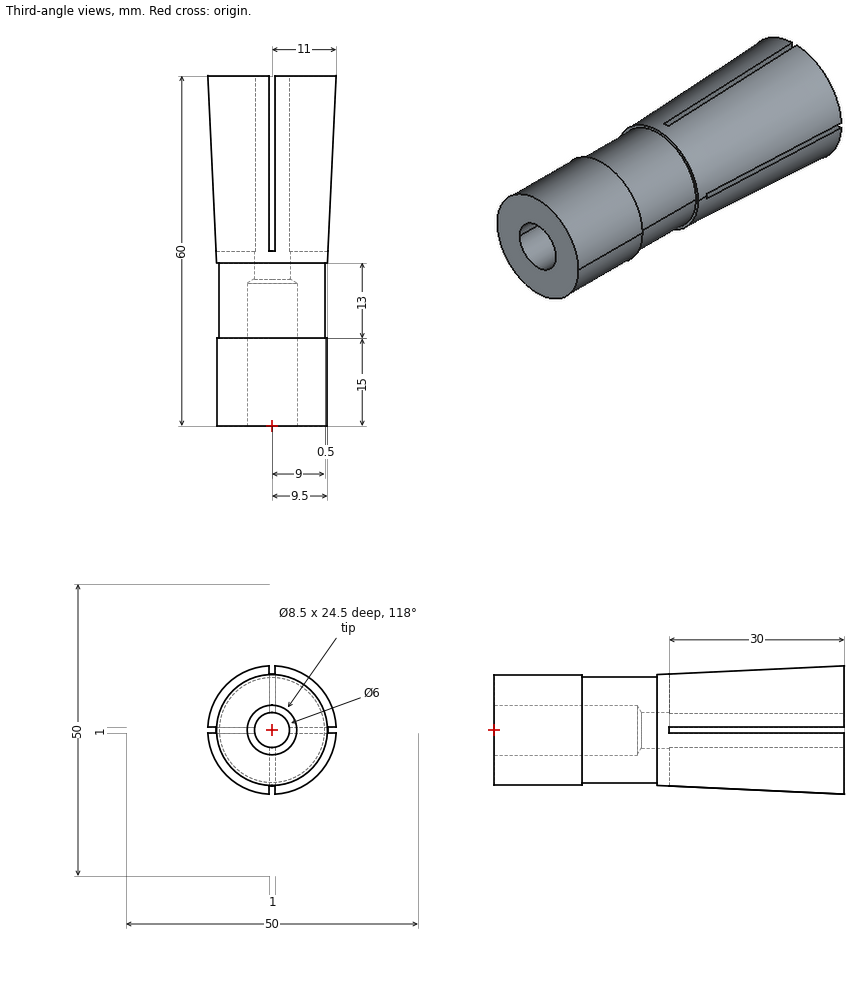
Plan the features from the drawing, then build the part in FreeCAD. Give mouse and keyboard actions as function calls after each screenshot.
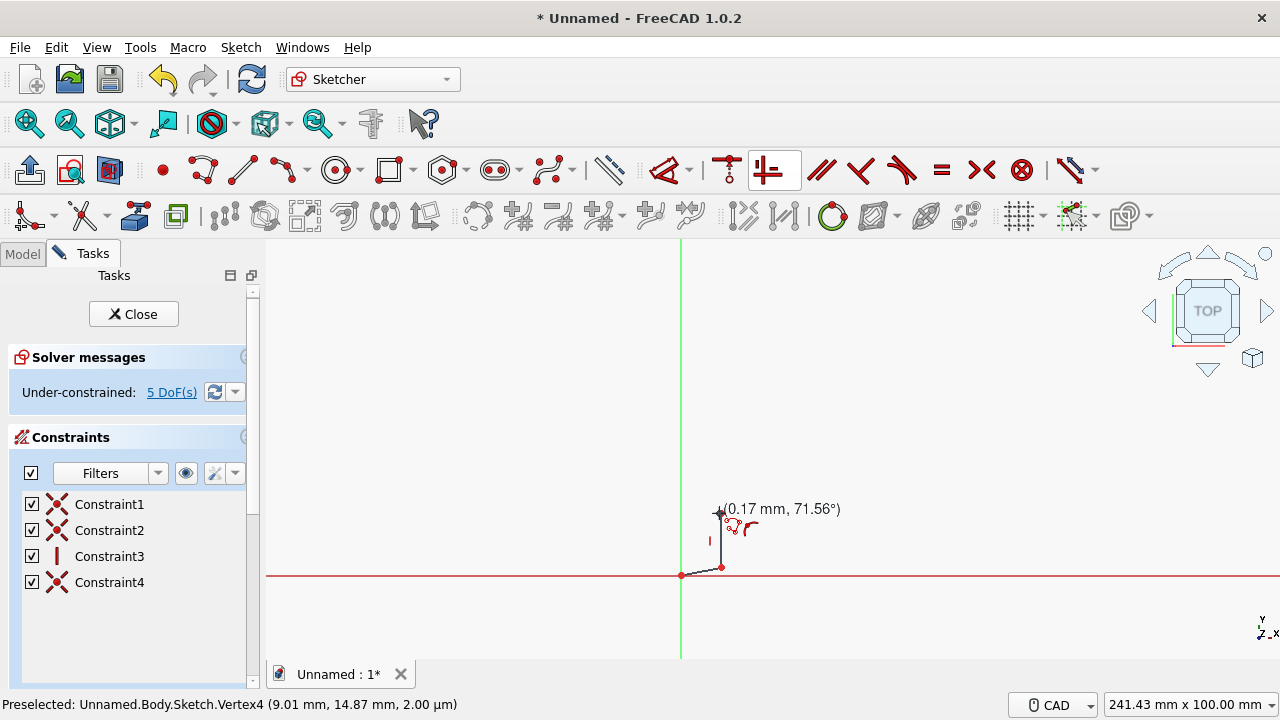
click(719, 458)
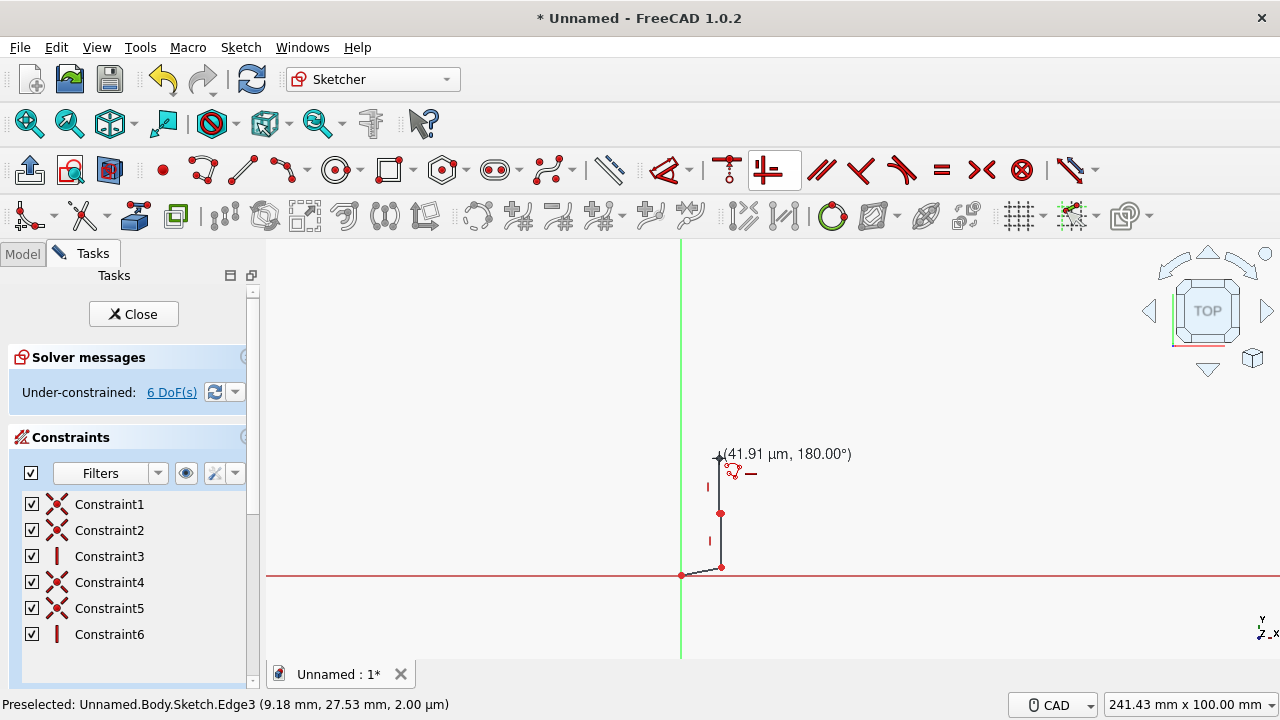
scroll(721, 458, up, 11)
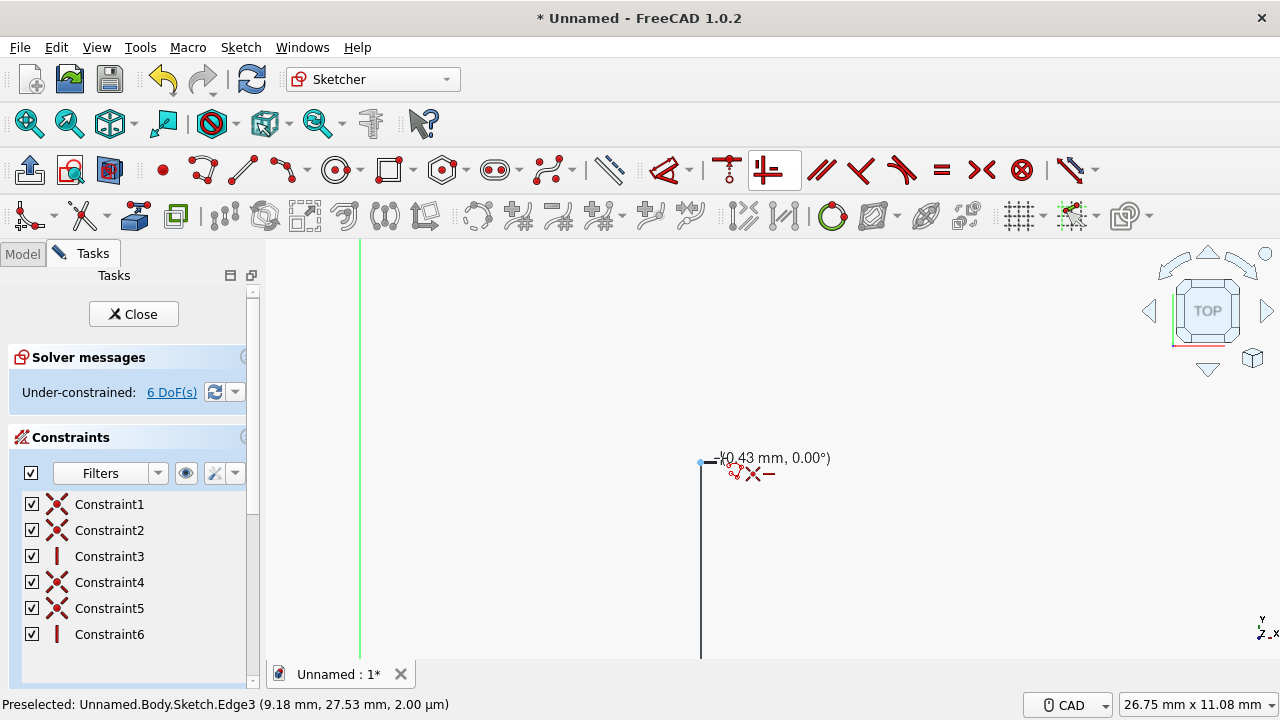
click(720, 454)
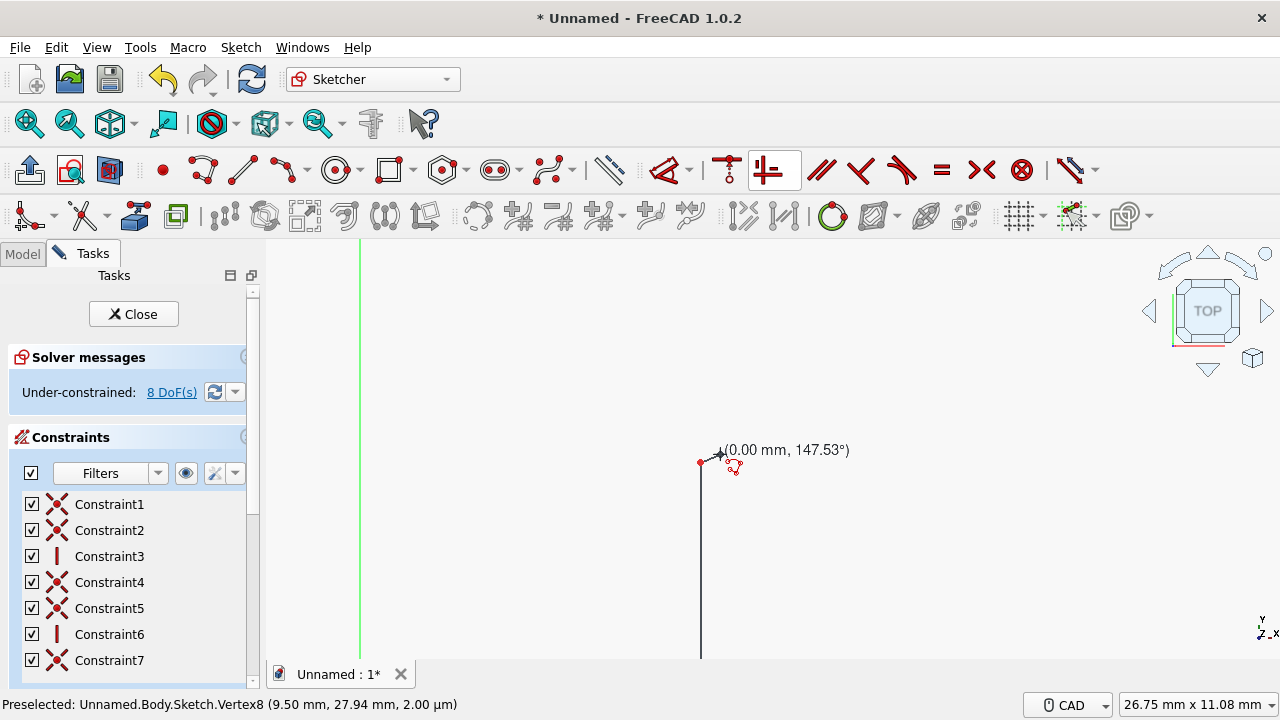
scroll(721, 458, down, 11)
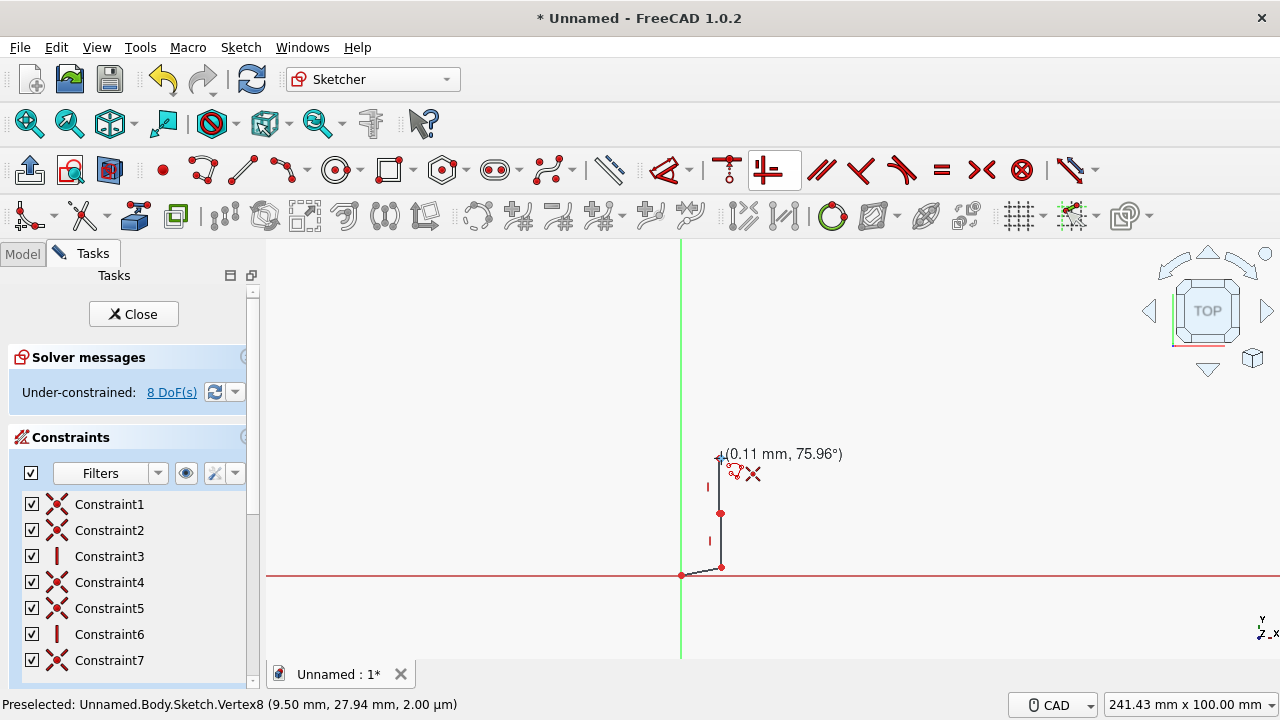
click(729, 324)
click(690, 324)
click(681, 576)
key(Escape)
key(Escape)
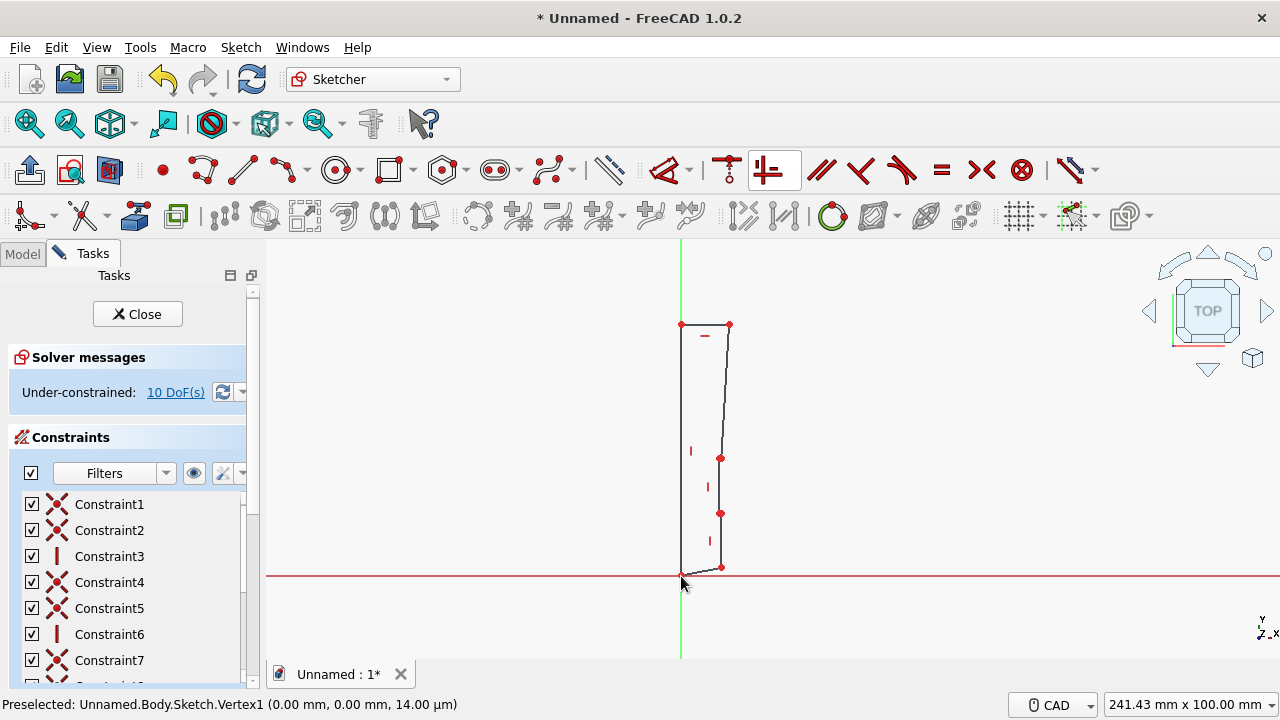
click(693, 573)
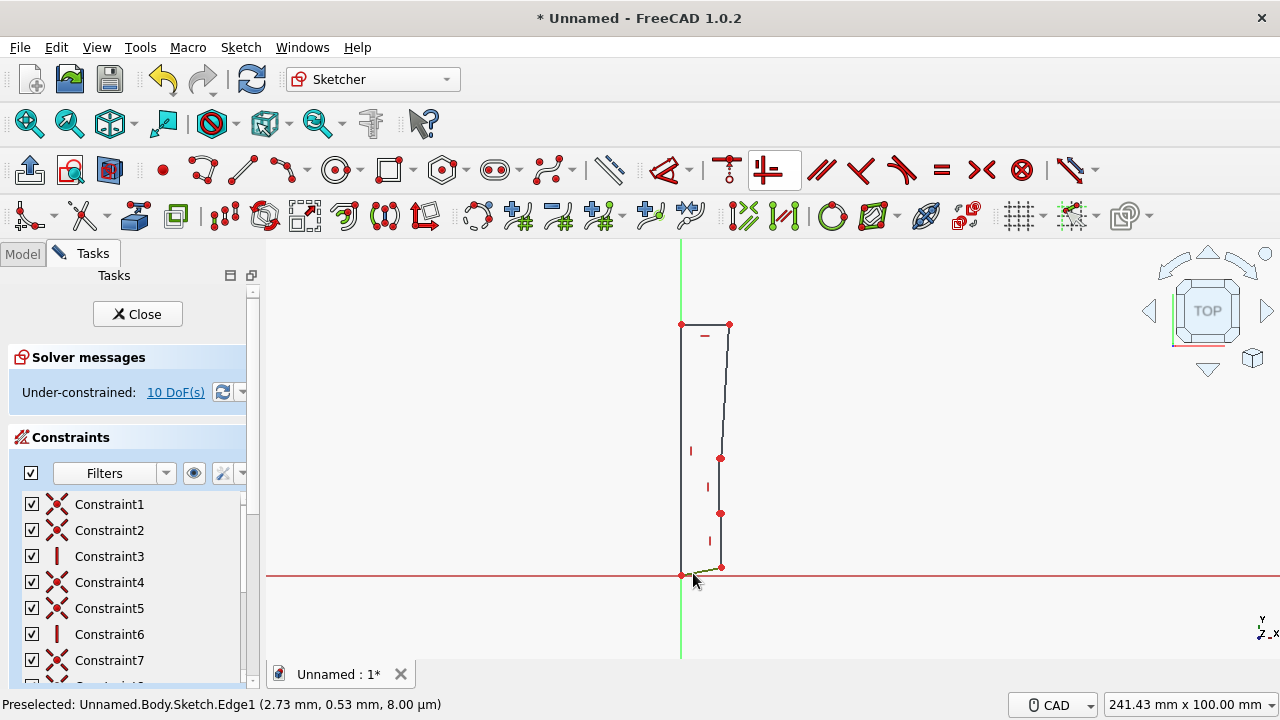
key(h)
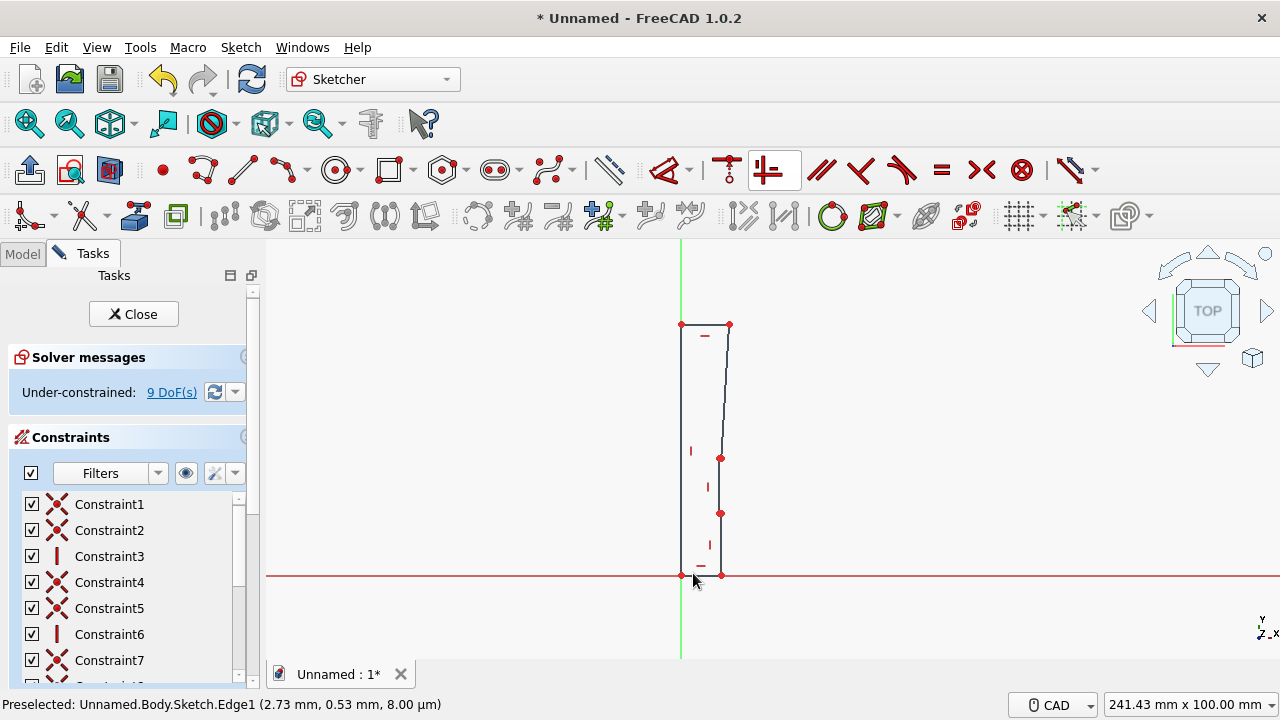
scroll(720, 513, up, 14)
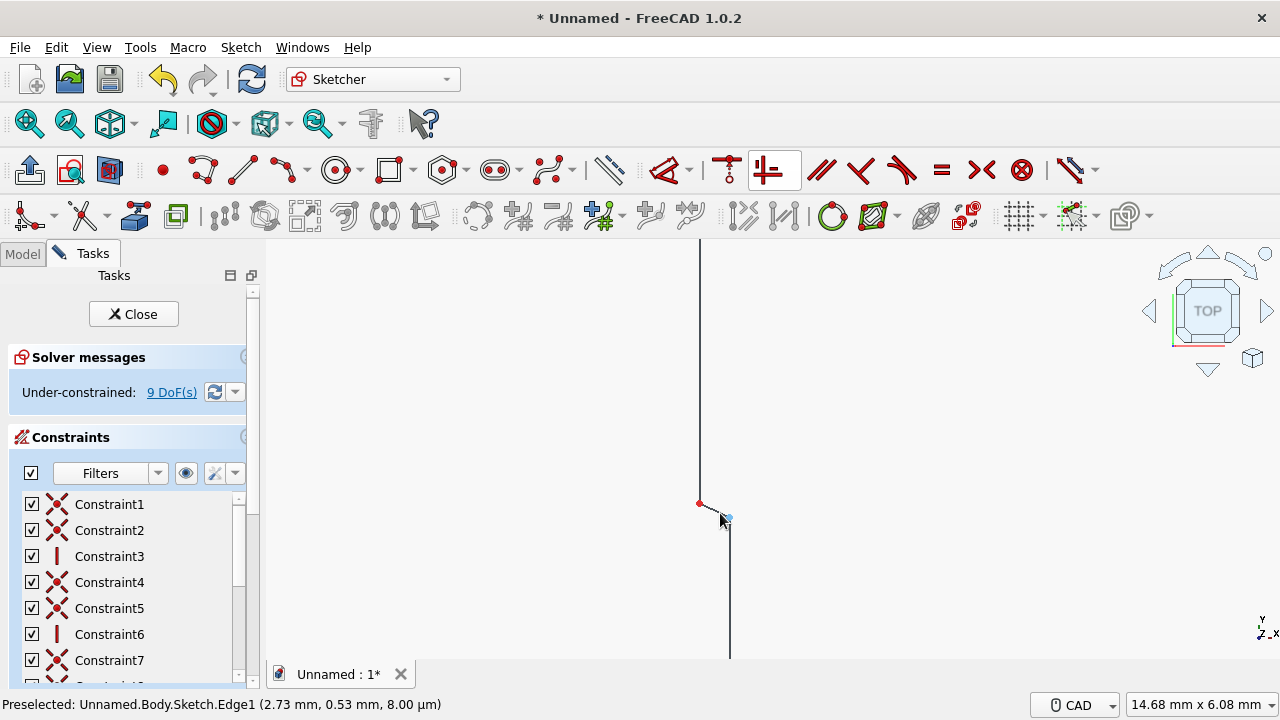
click(715, 510)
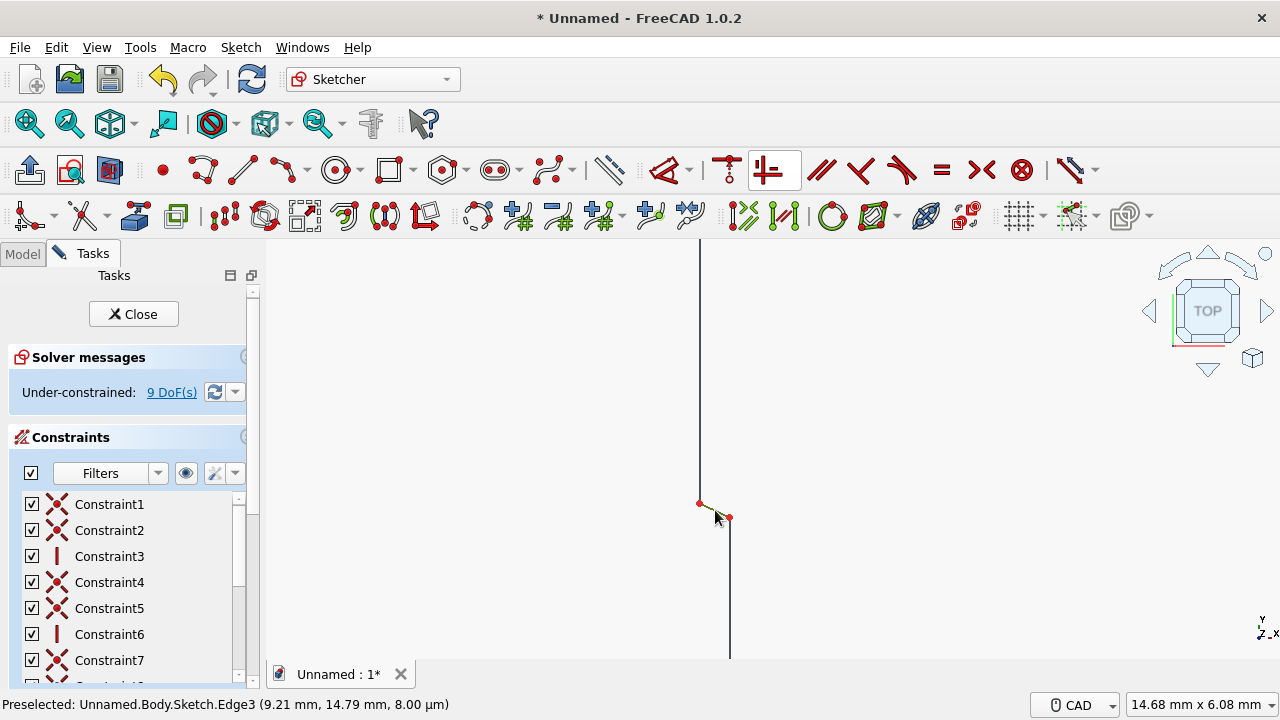
click(796, 170)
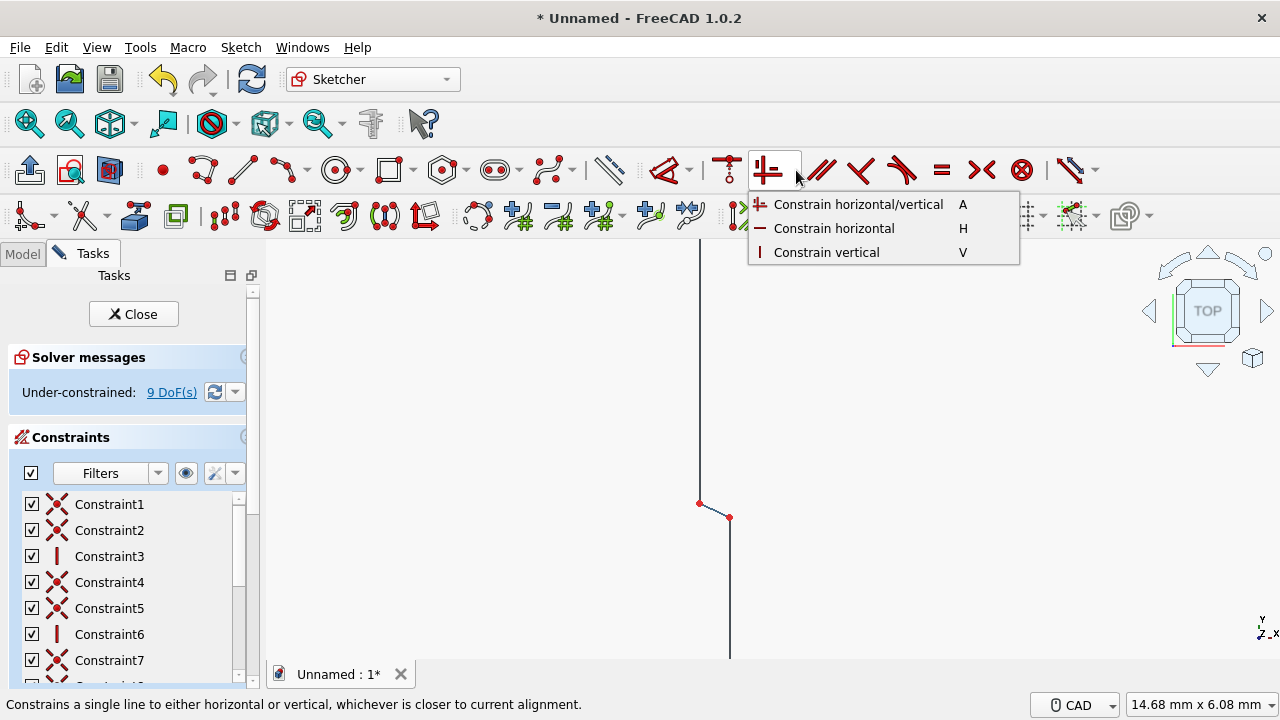
click(884, 228)